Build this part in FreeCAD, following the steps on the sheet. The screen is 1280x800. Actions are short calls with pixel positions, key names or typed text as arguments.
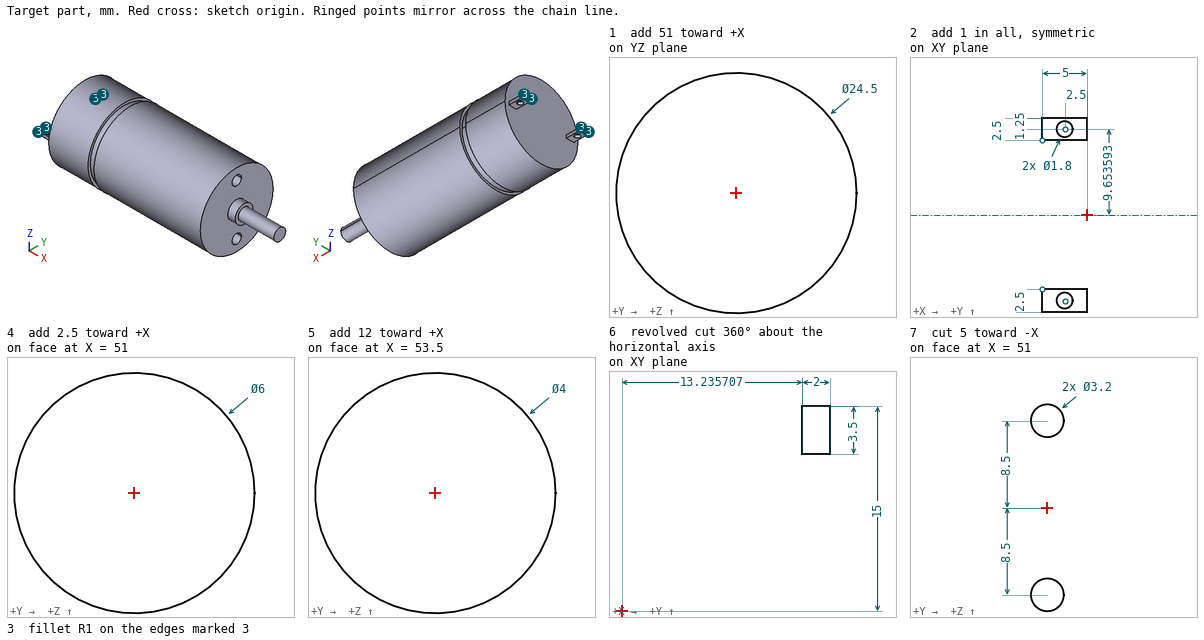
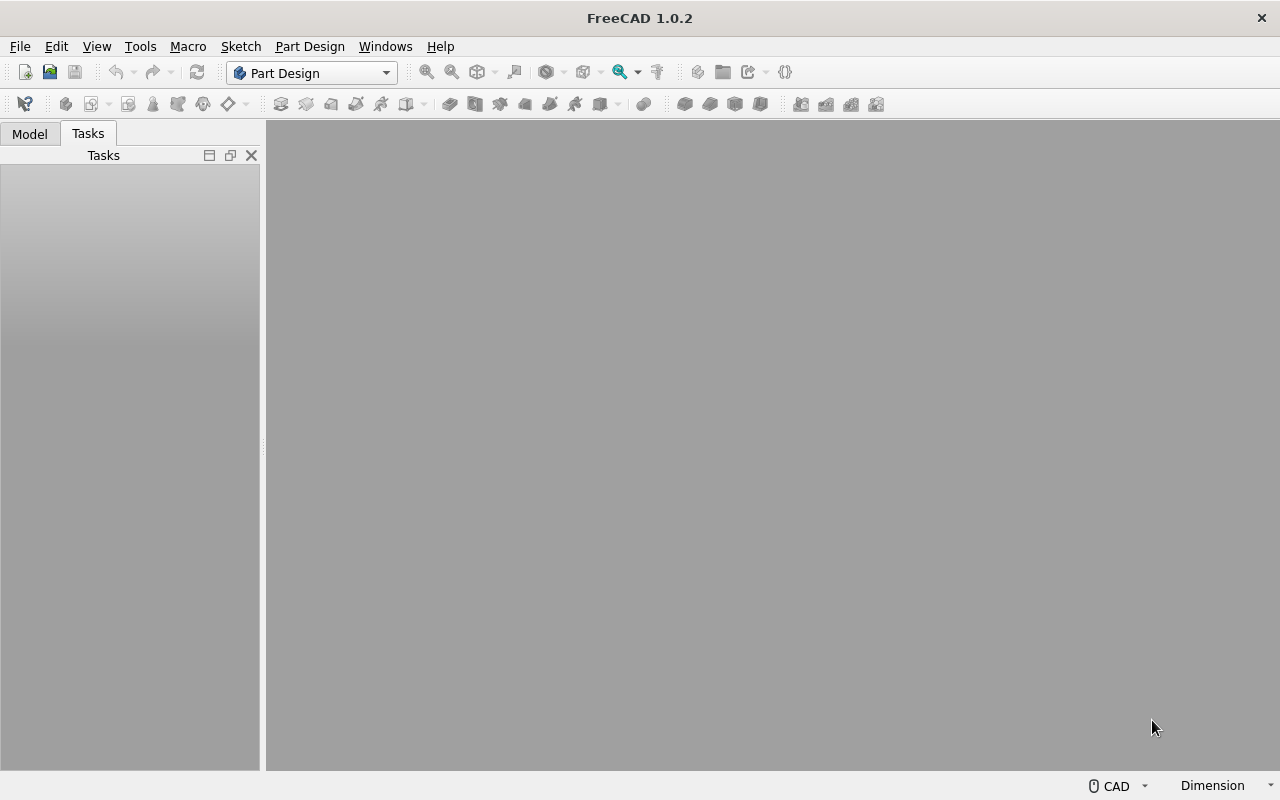
click(25, 72)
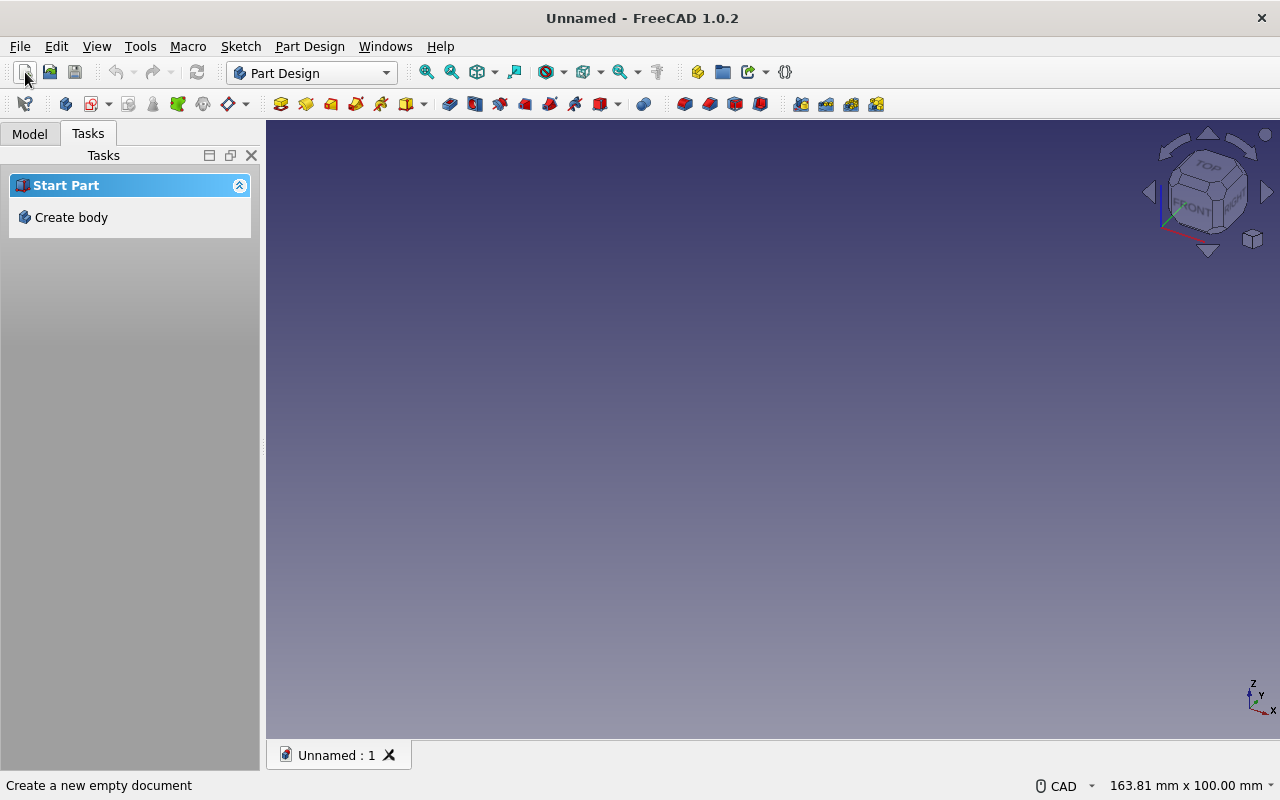
click(90, 104)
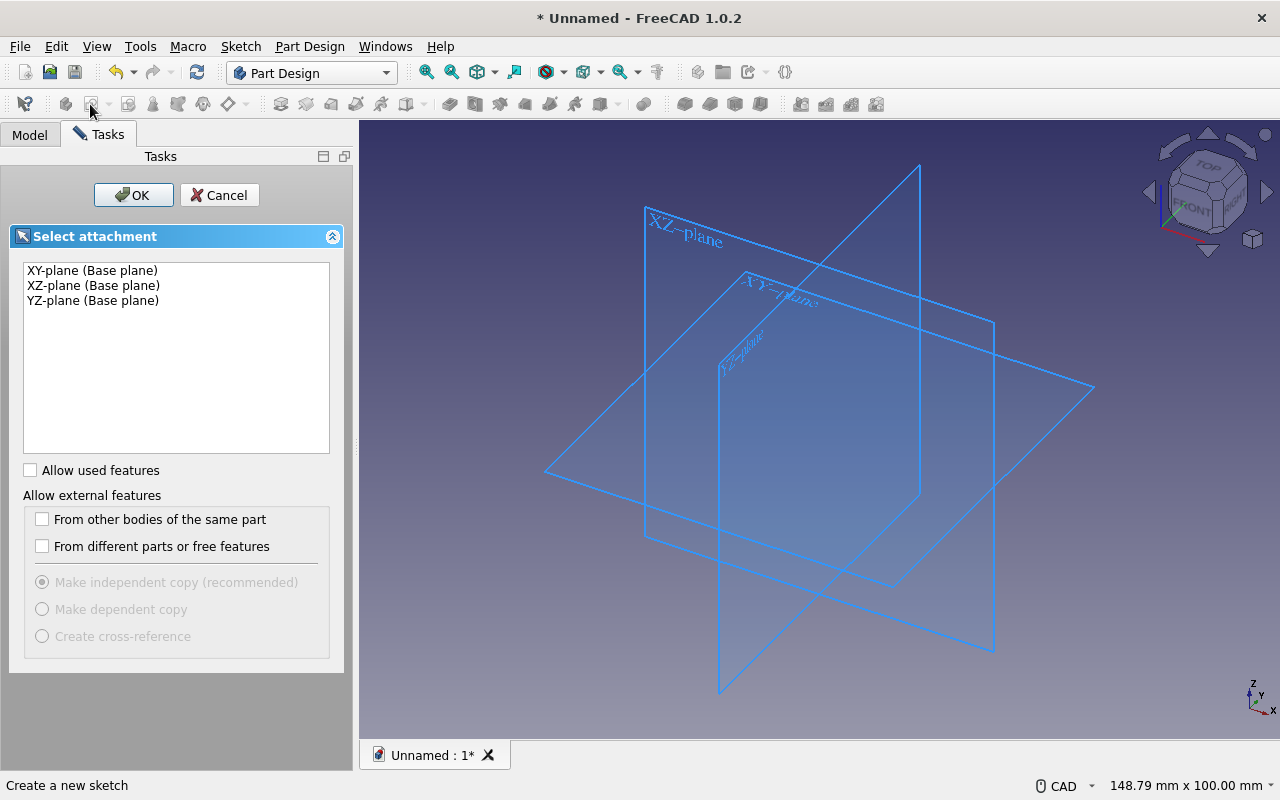
click(84, 300)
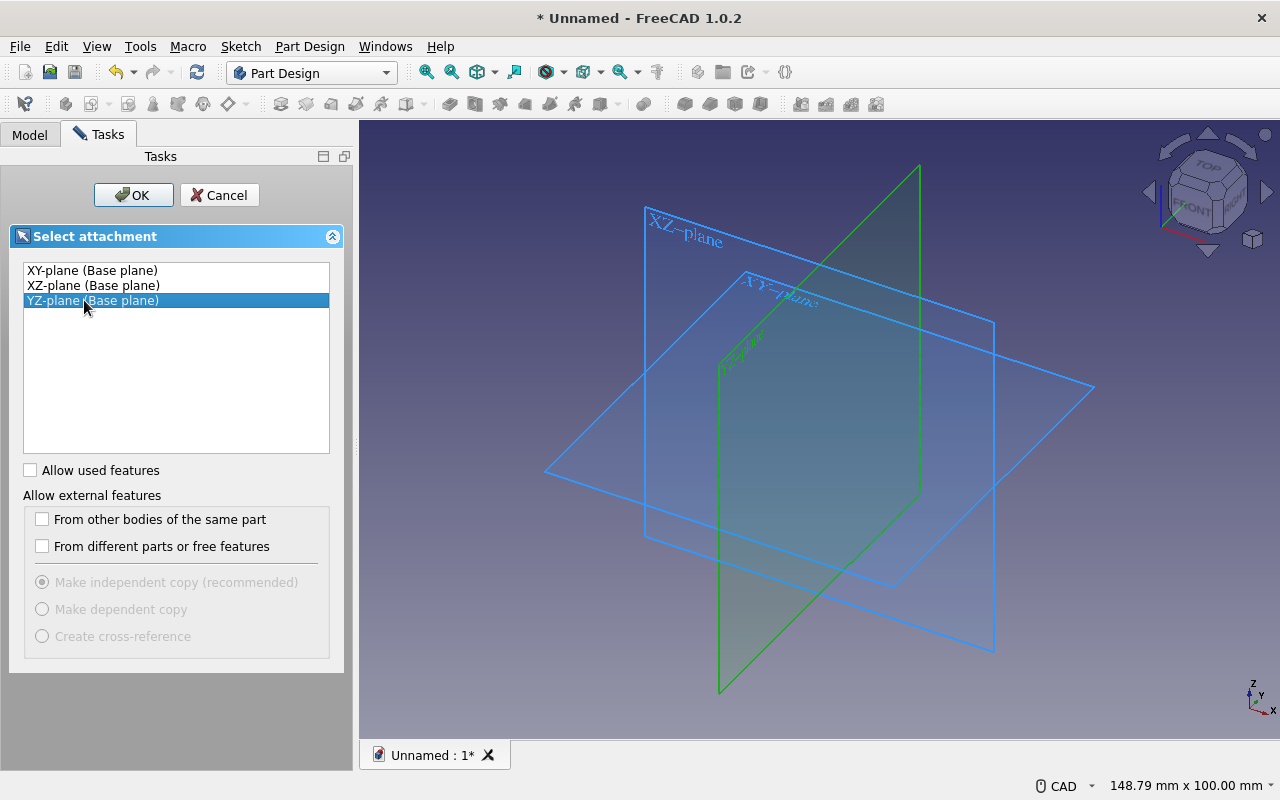
click(134, 195)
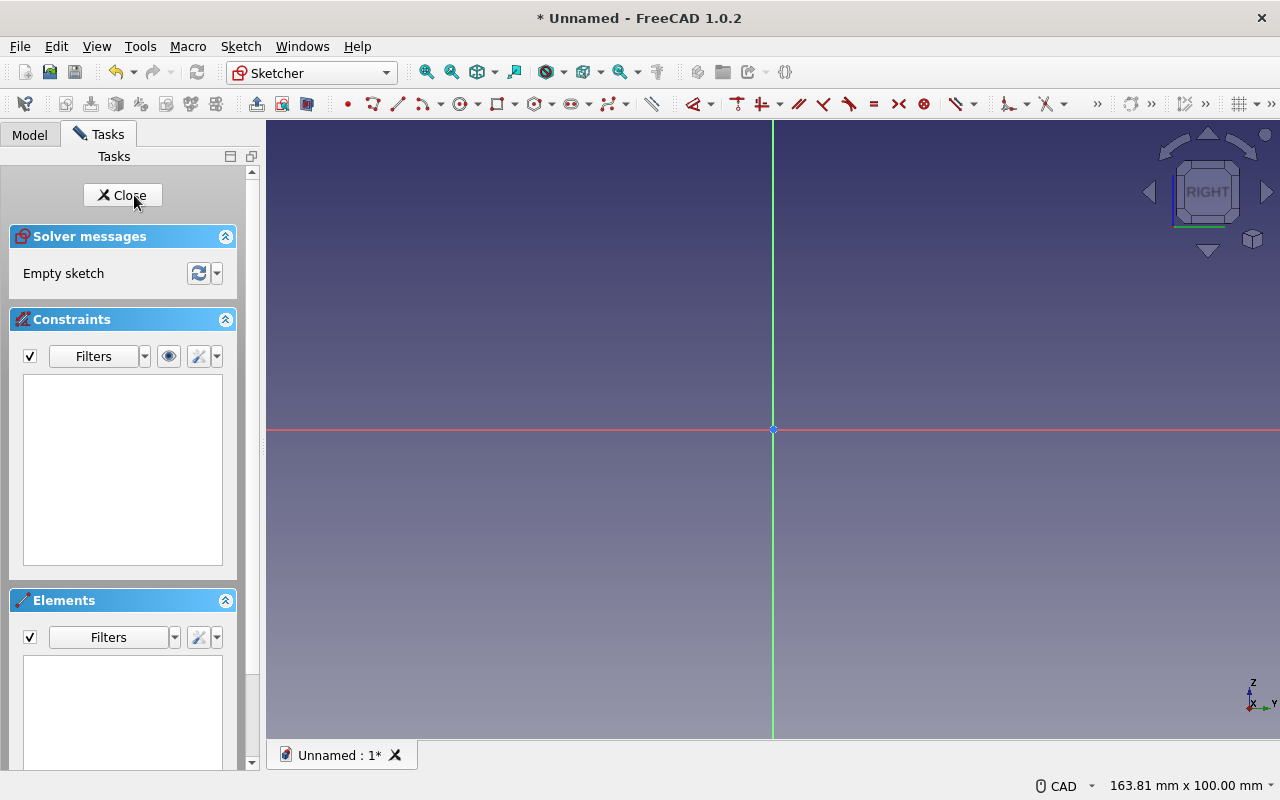
scroll(813, 429, up, 5)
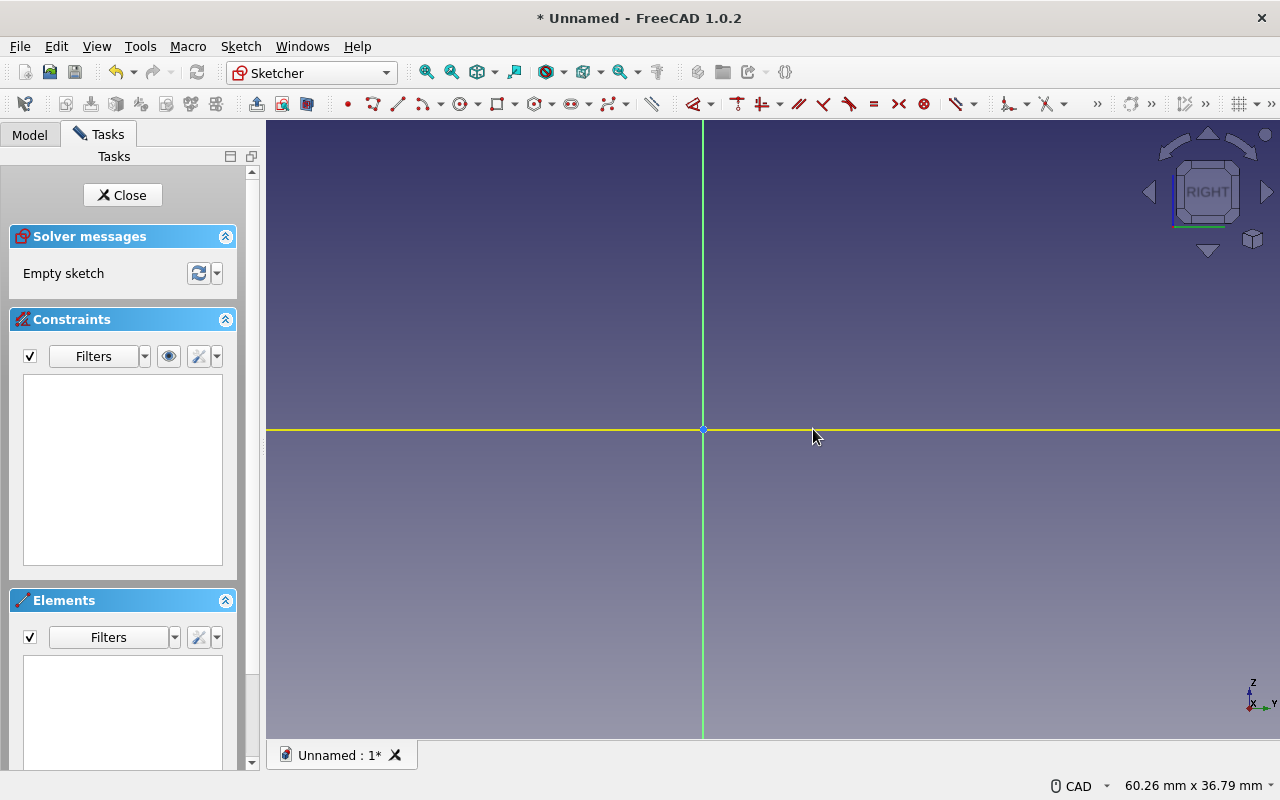
click(460, 104)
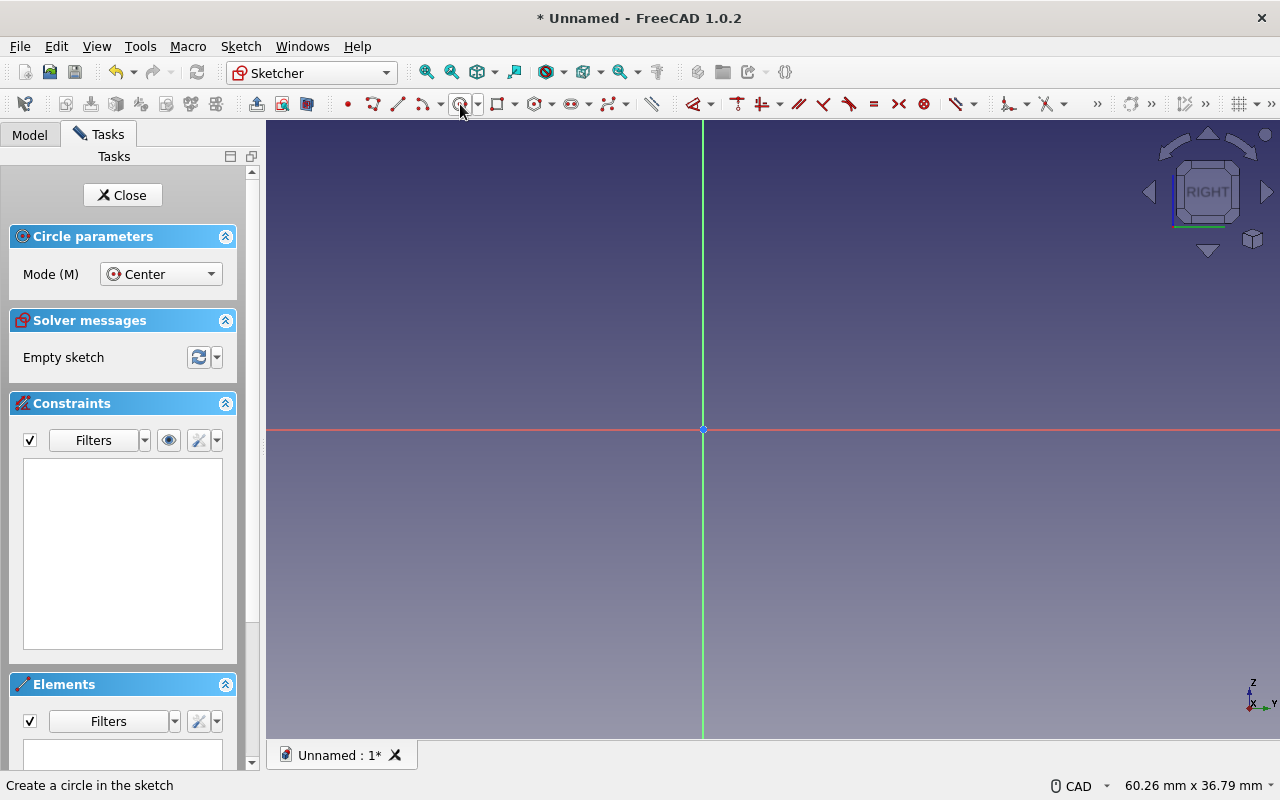
click(703, 430)
move(849, 284)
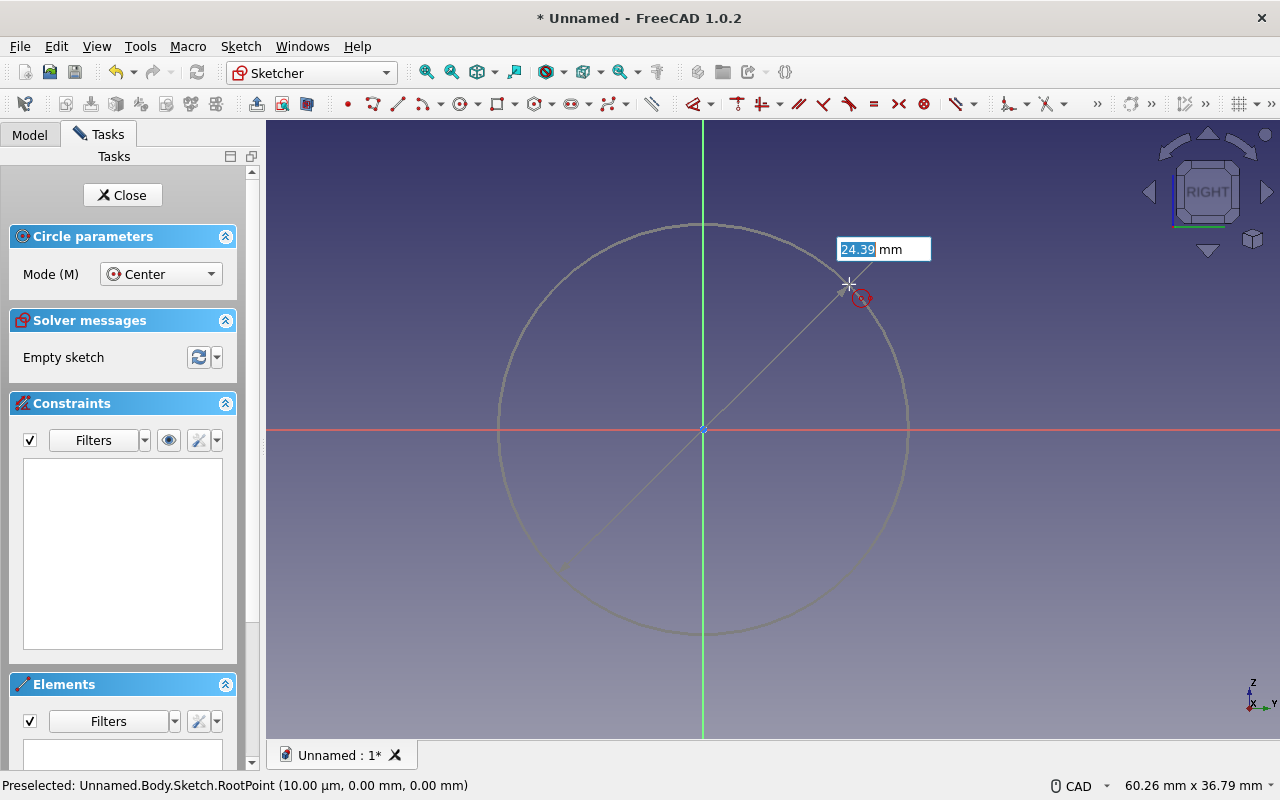
text(24.5)
key(Return)
key(Escape)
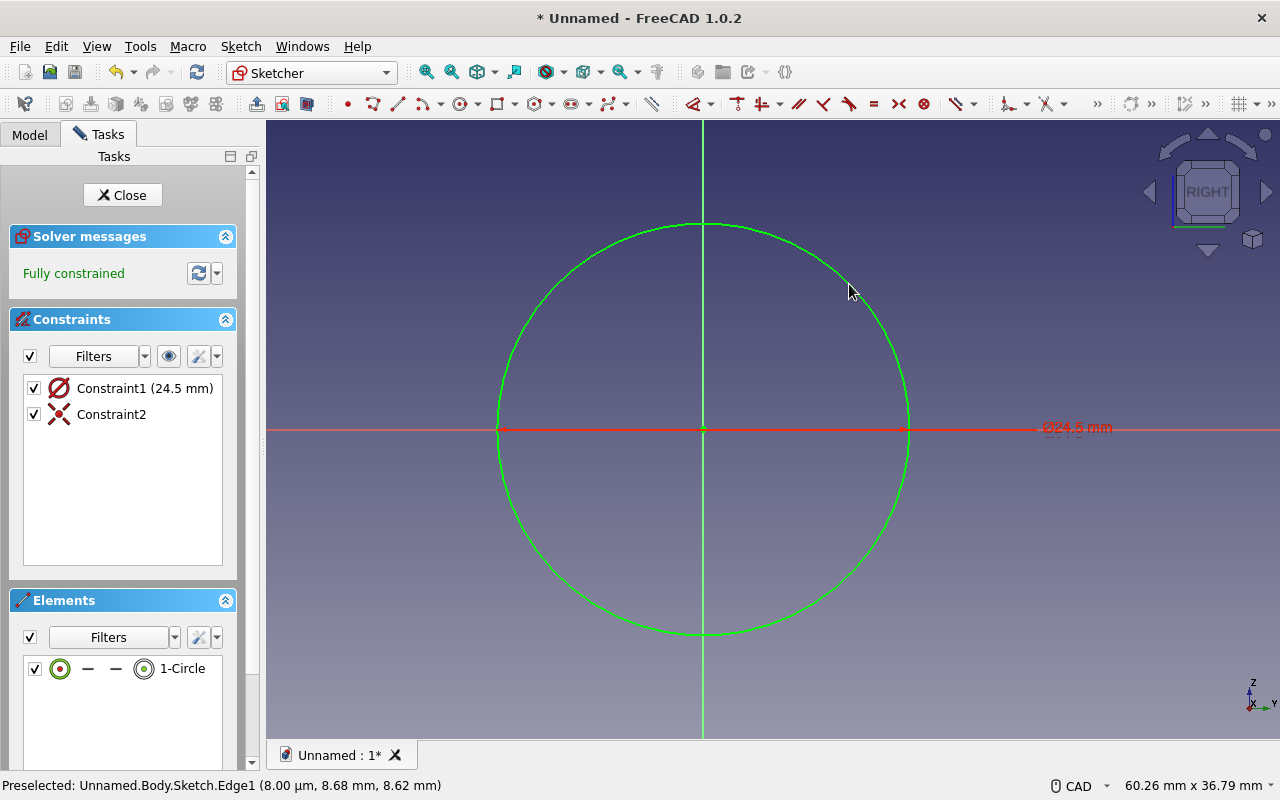
click(123, 195)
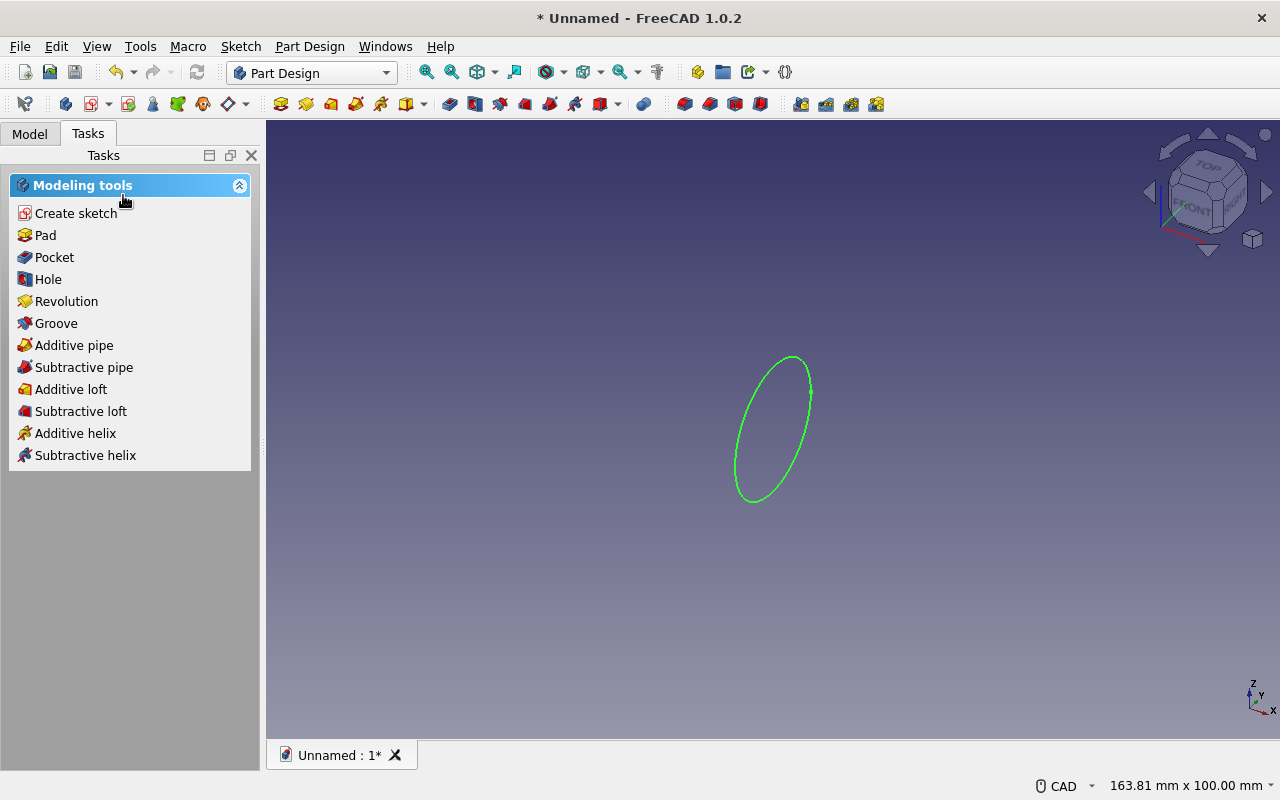
click(281, 104)